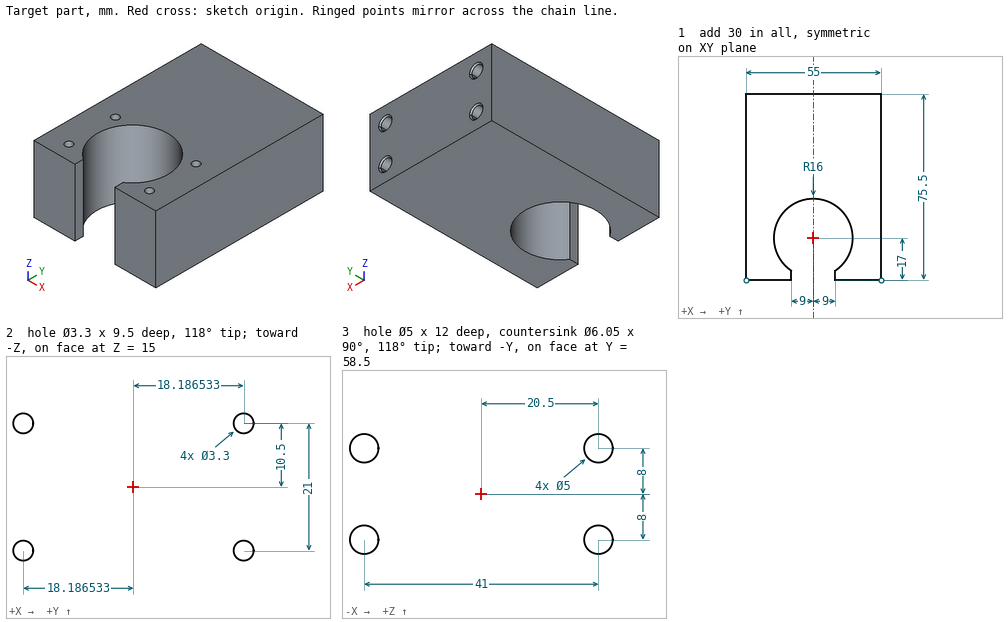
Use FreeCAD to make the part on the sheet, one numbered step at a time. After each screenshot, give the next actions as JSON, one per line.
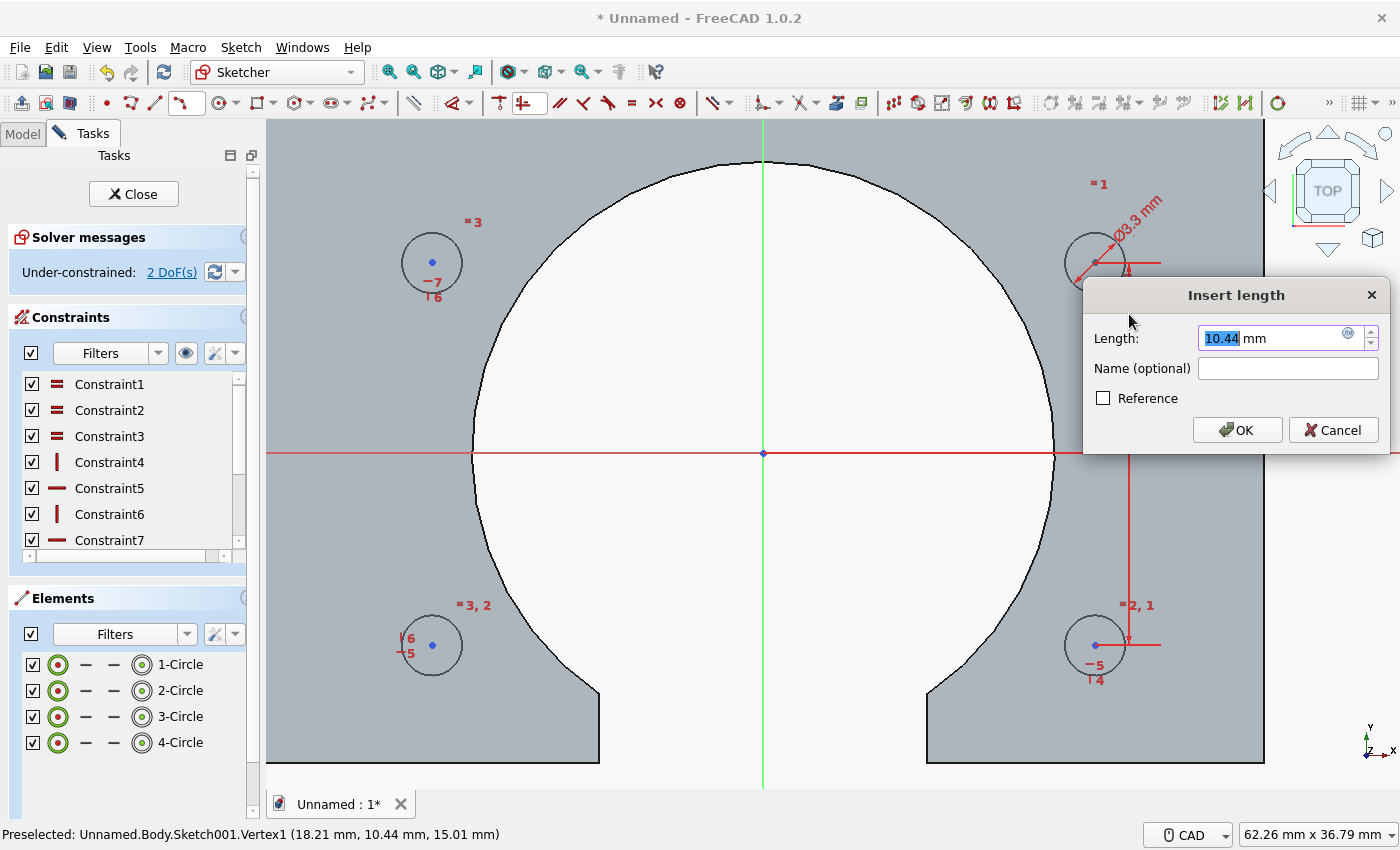
{"action": "type", "text": "10.5"}
{"action": "key", "text": "Return"}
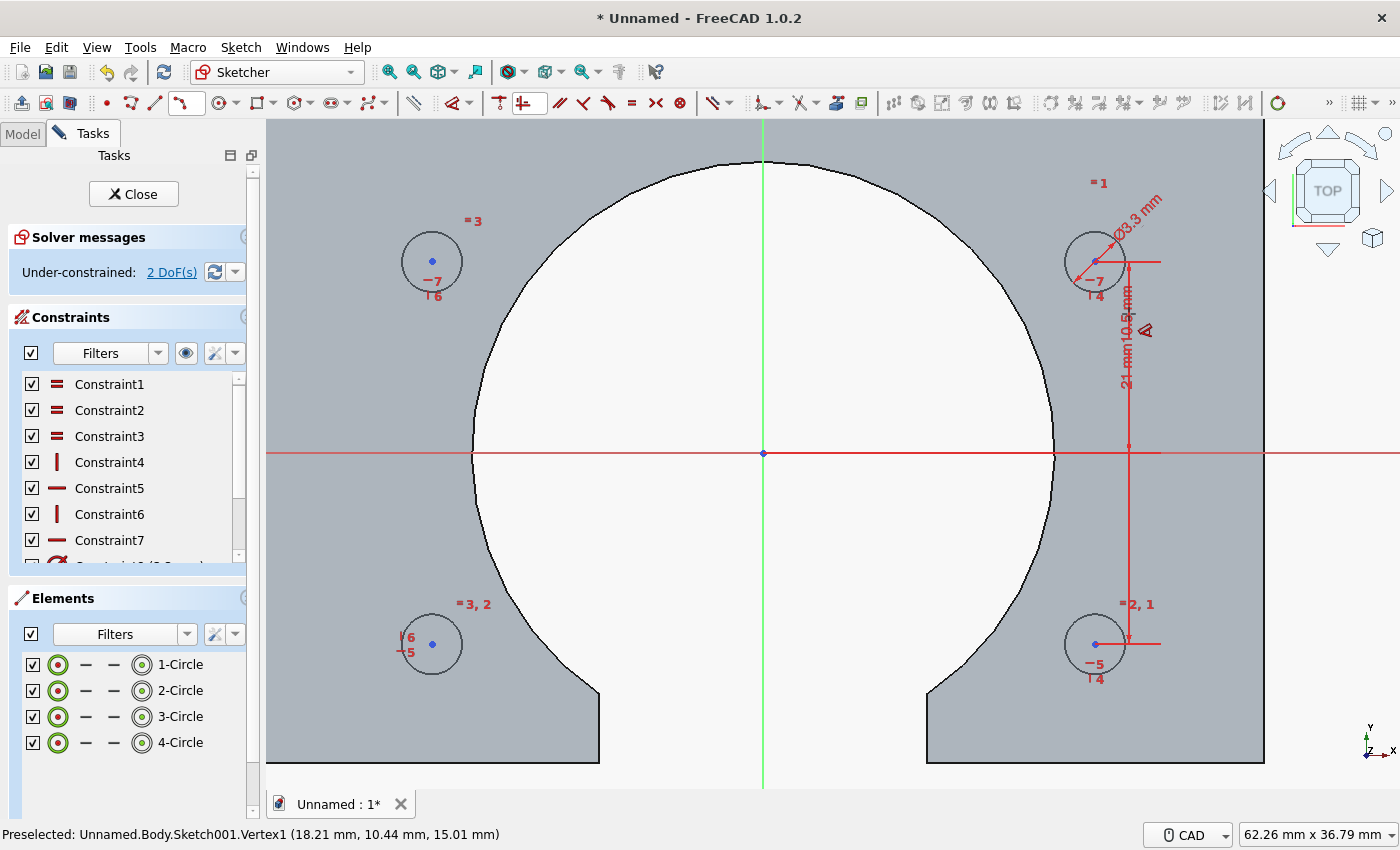
{"action": "left_click", "coordinate": [1095, 262]}
{"action": "left_click", "coordinate": [929, 228]}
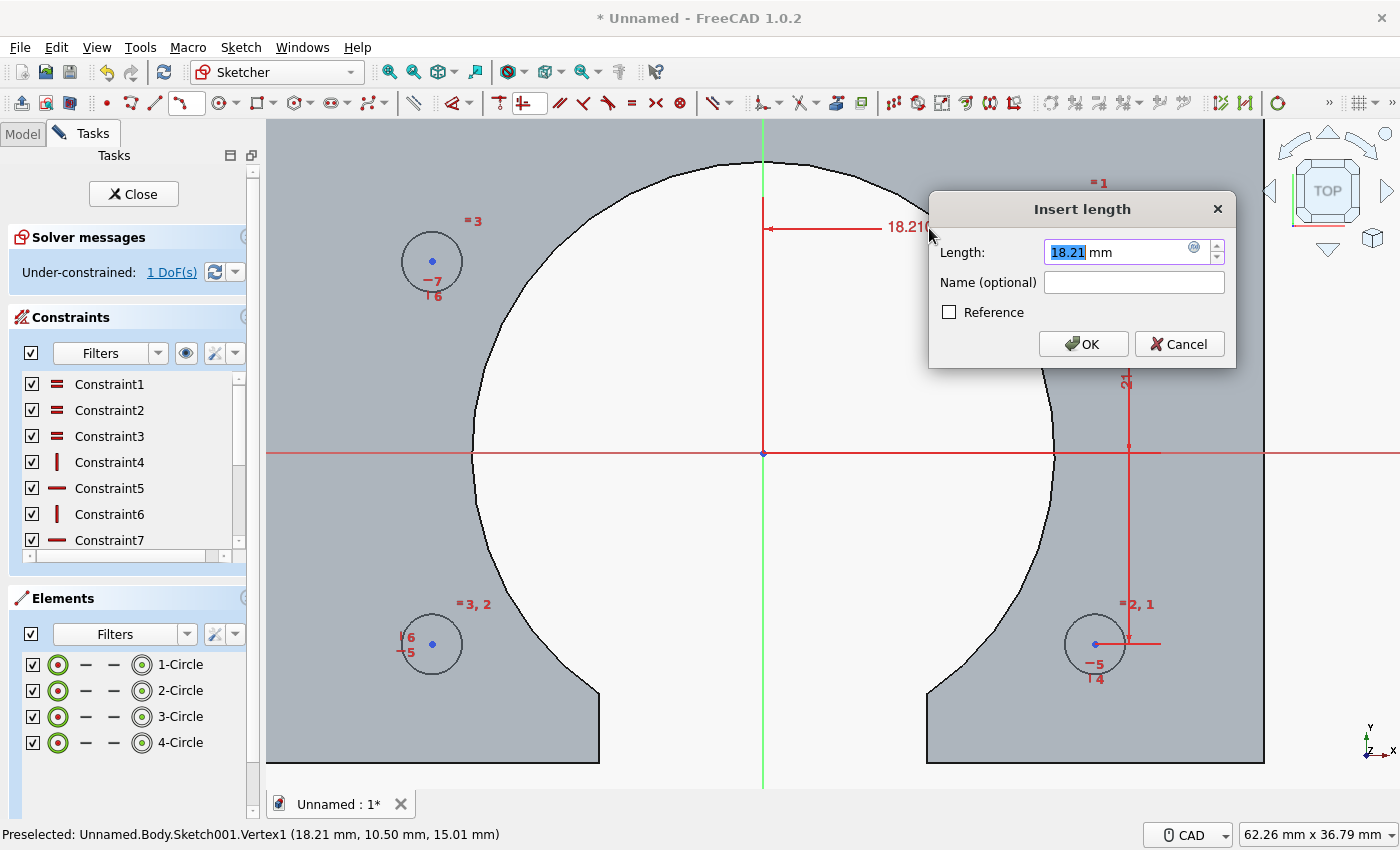
{"action": "type", "text": "18.186533"}
{"action": "key", "text": "Return"}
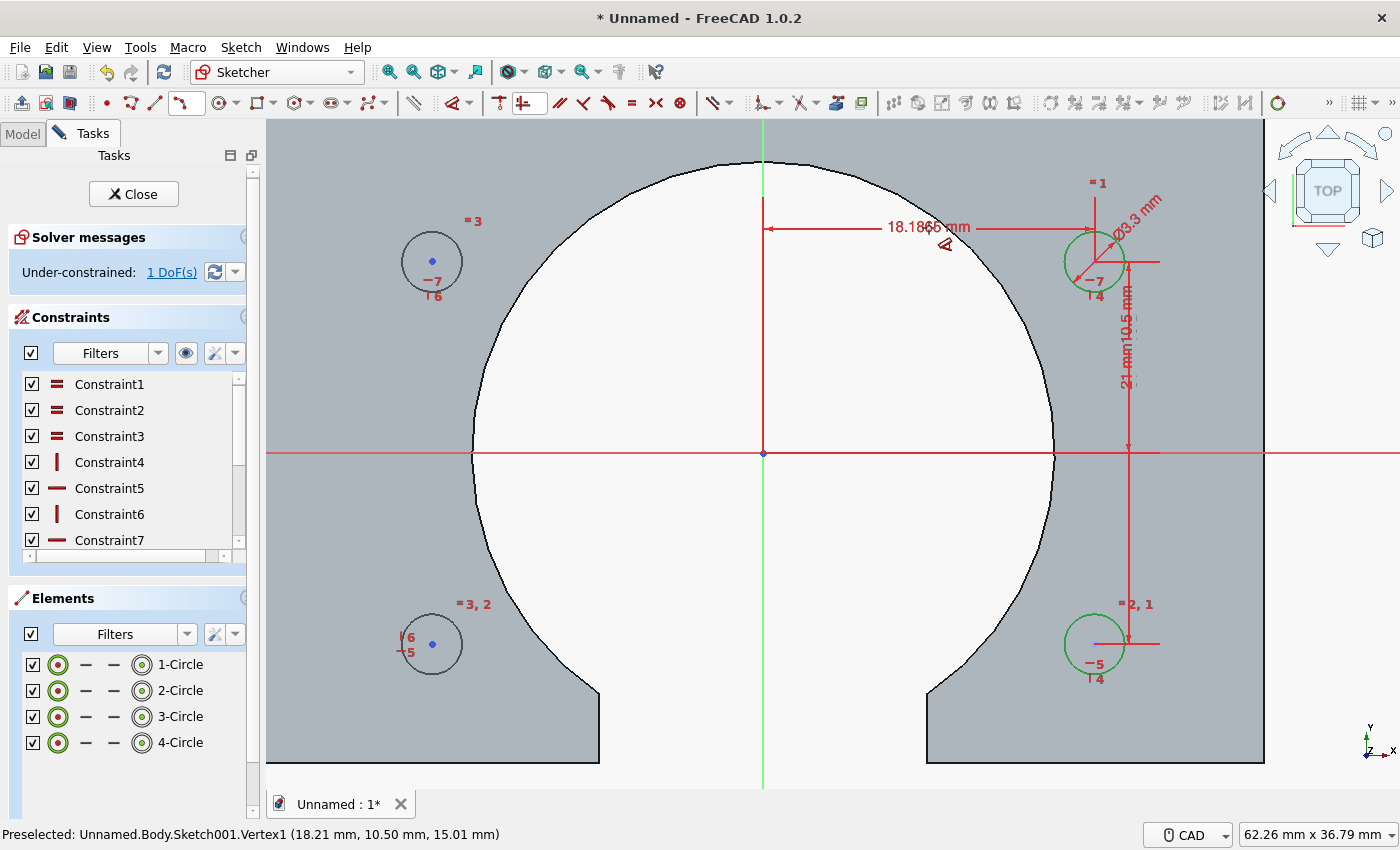
{"action": "left_click", "coordinate": [432, 644]}
{"action": "left_click", "coordinate": [598, 678]}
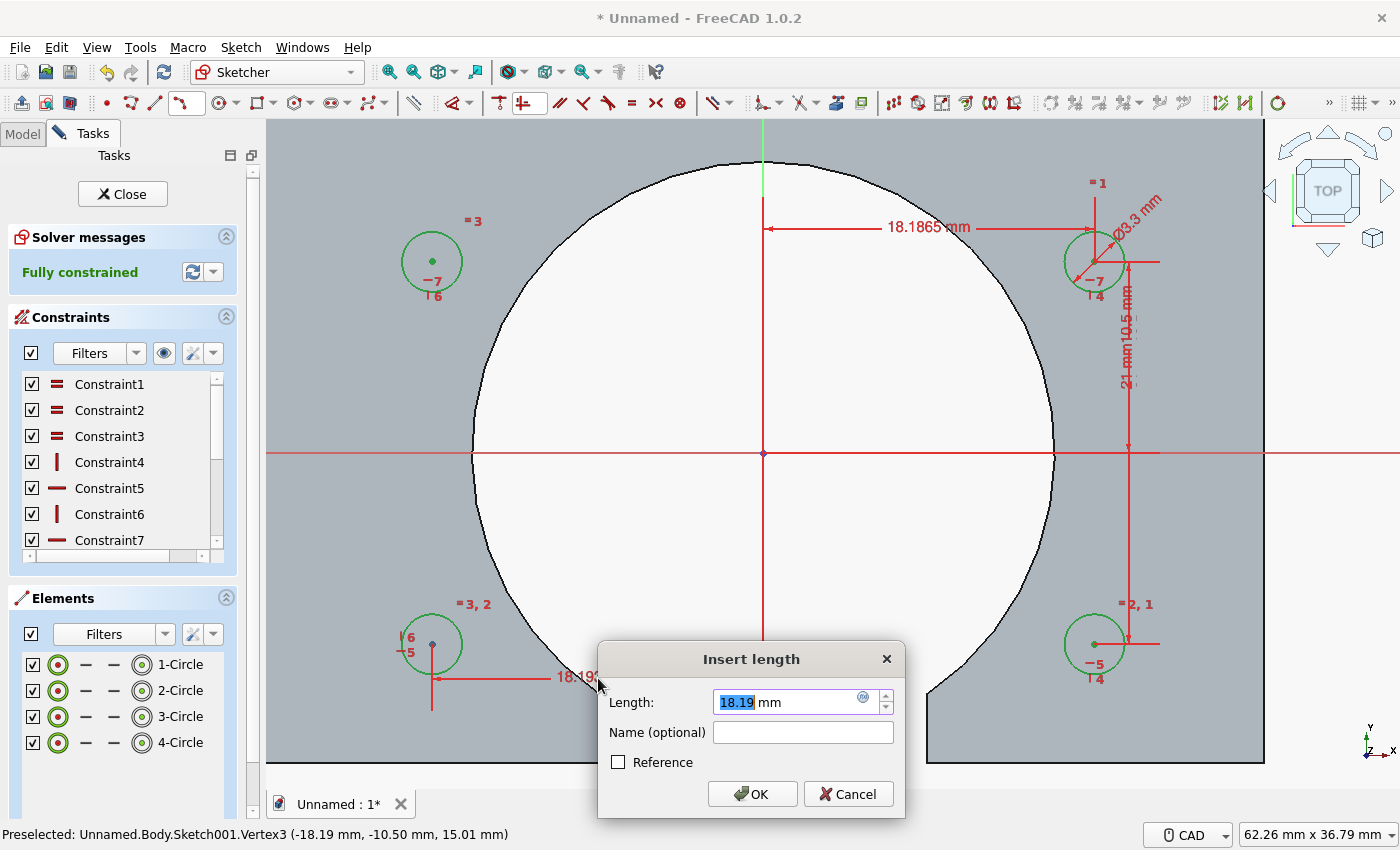
{"action": "type", "text": "18.186533"}
{"action": "key", "text": "Return"}
{"action": "key", "text": "Escape"}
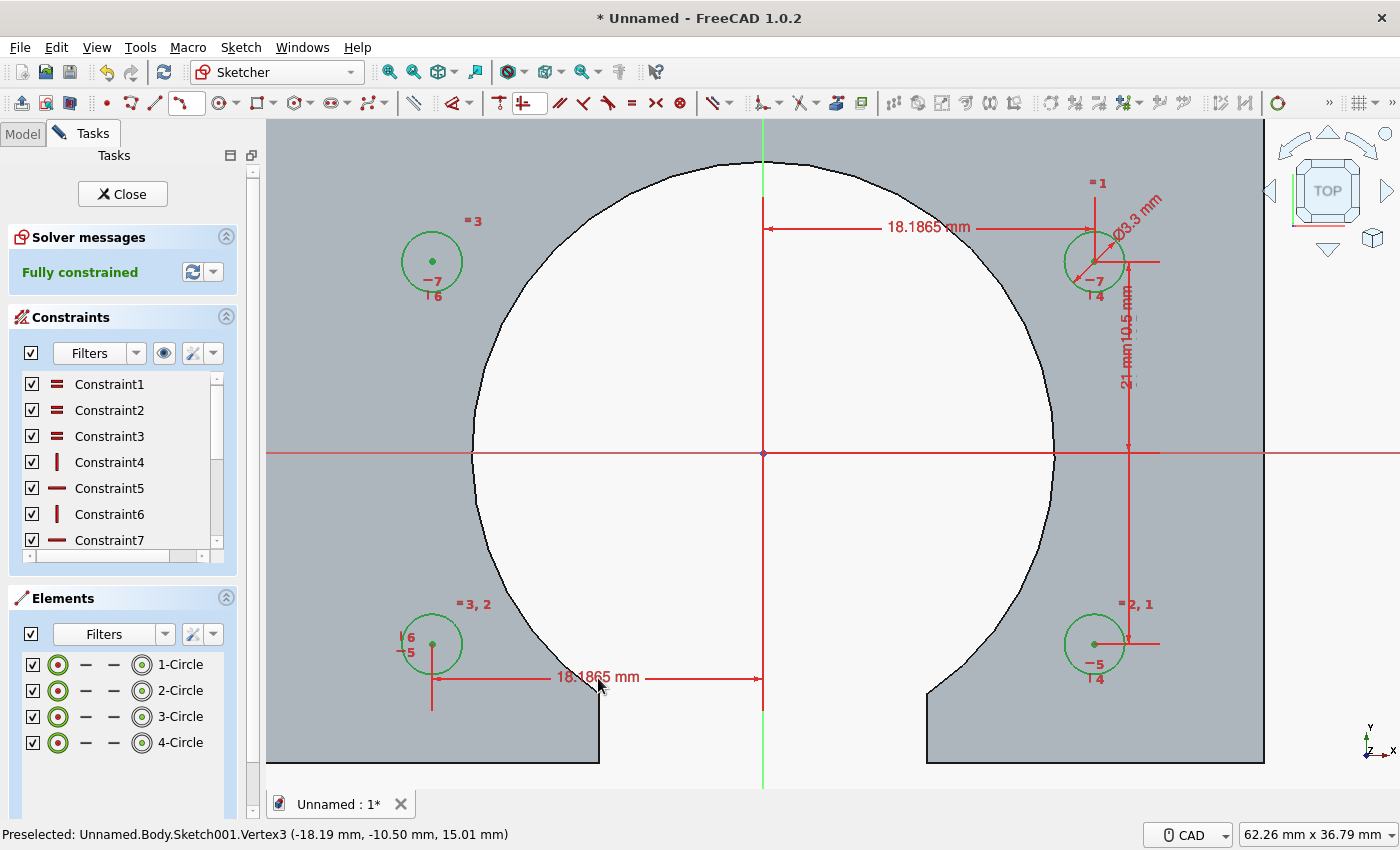
{"action": "left_click", "coordinate": [123, 194]}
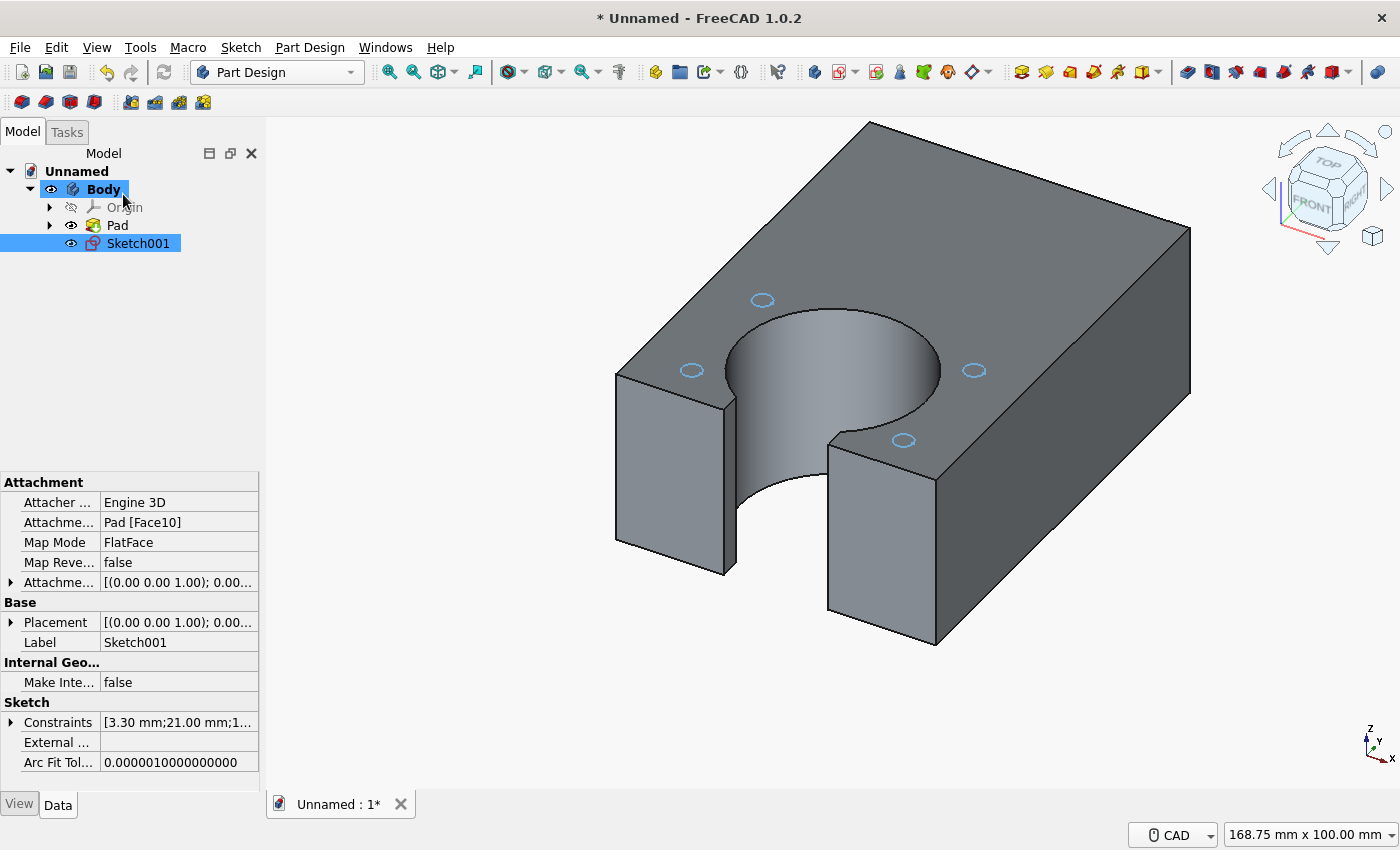
{"action": "left_click", "coordinate": [1212, 72]}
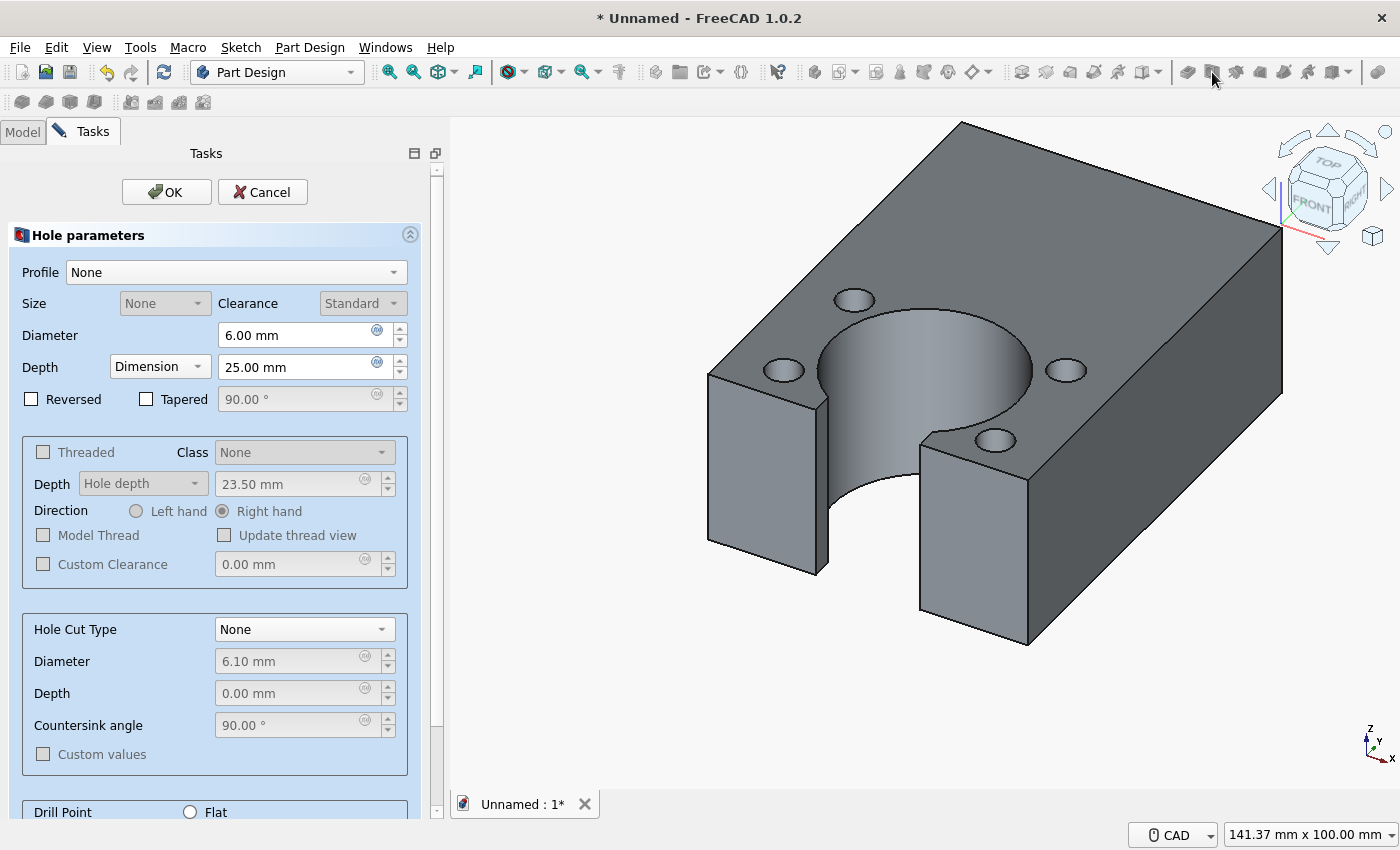
{"action": "triple_click", "coordinate": [305, 335]}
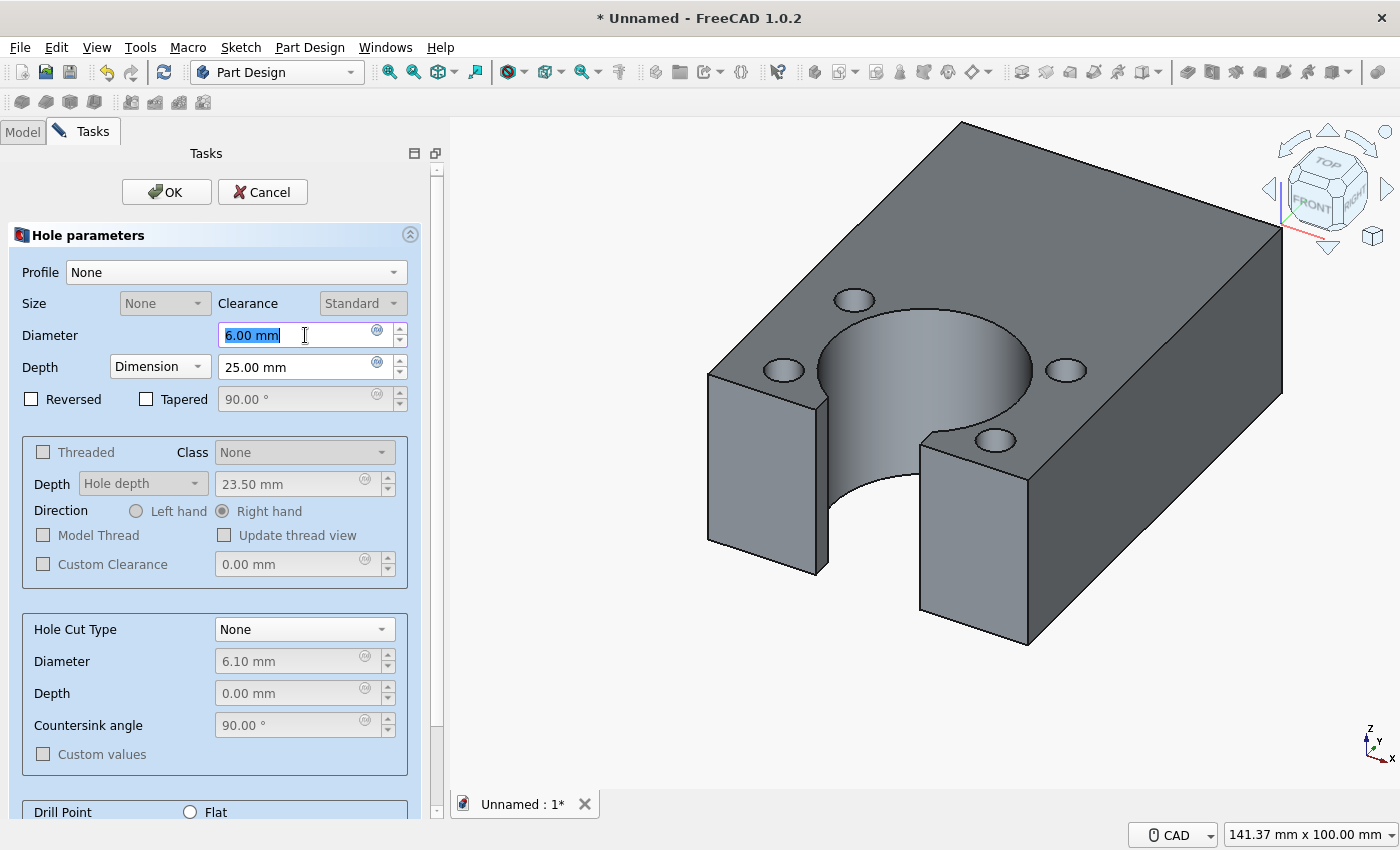
{"action": "type", "text": "3.3"}
{"action": "key", "text": "Tab"}